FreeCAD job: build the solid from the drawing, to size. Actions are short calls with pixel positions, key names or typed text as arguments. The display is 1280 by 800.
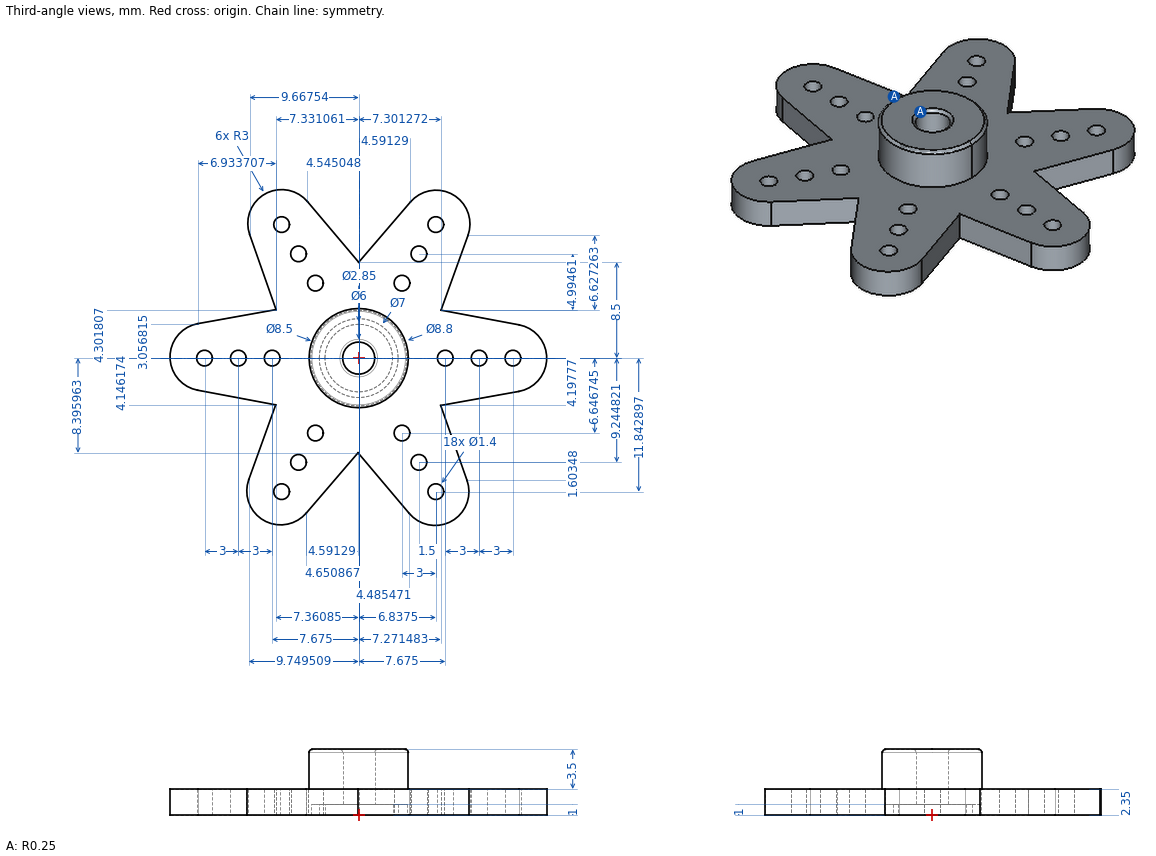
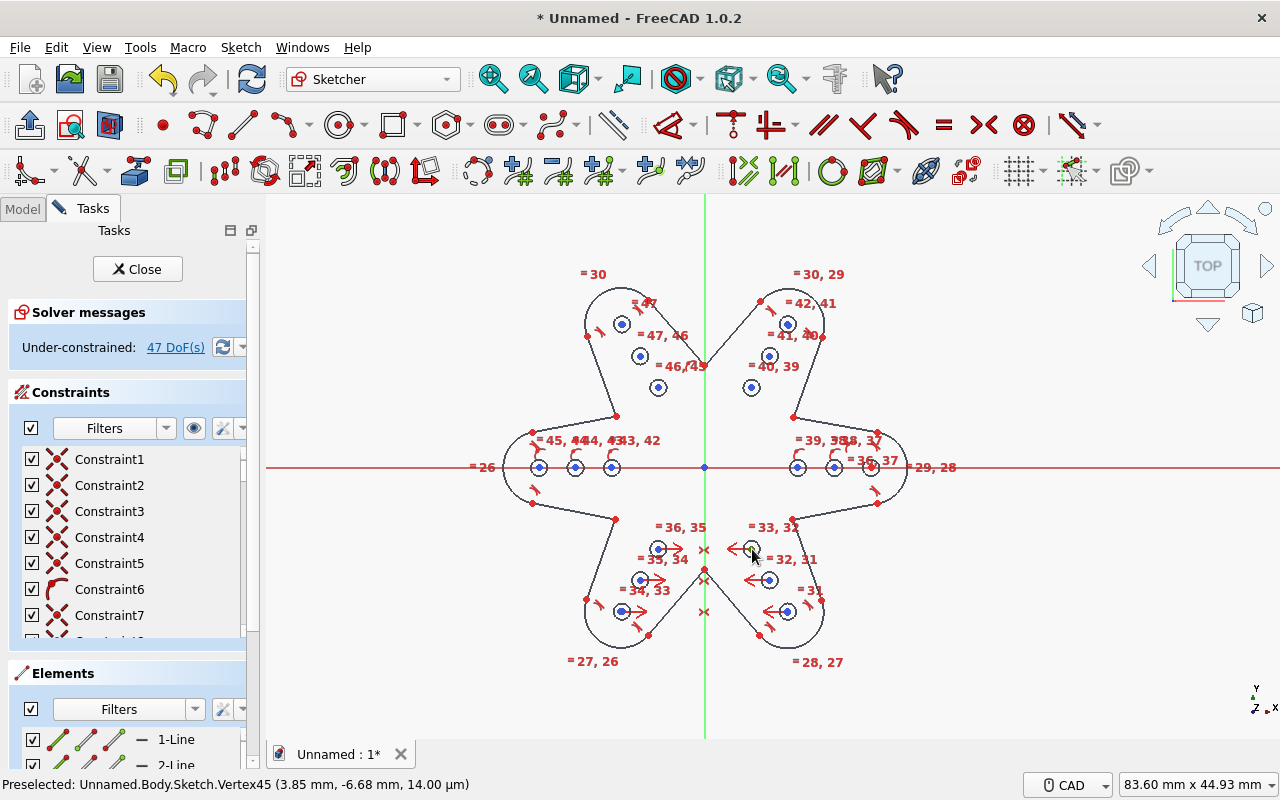
click(752, 388)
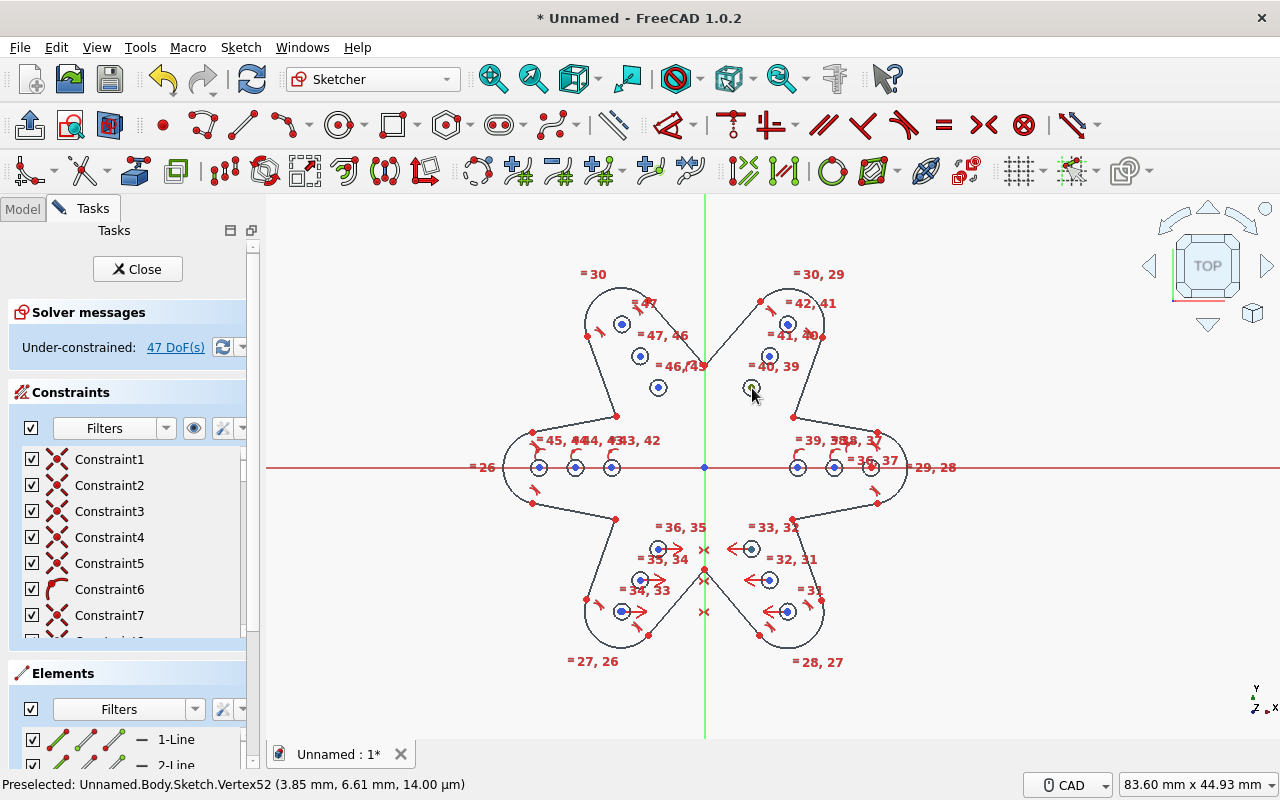
click(353, 468)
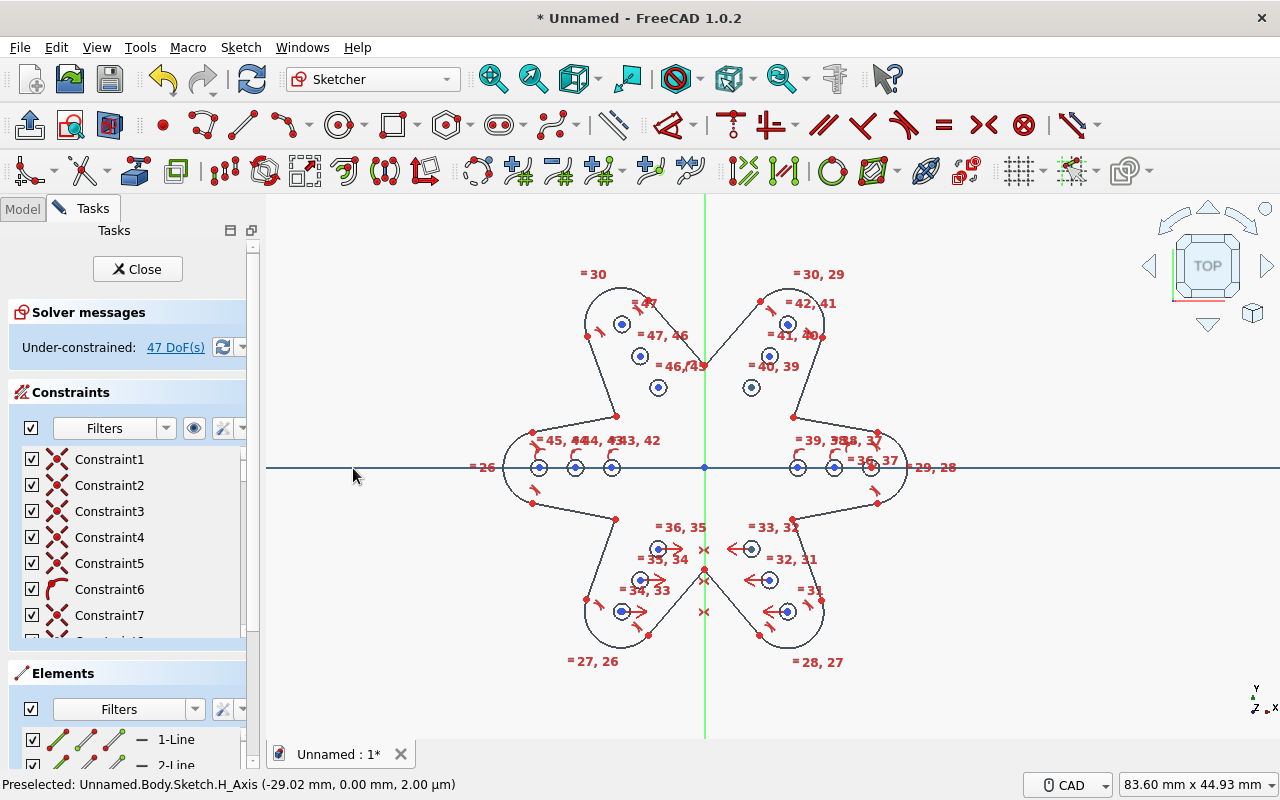
click(984, 126)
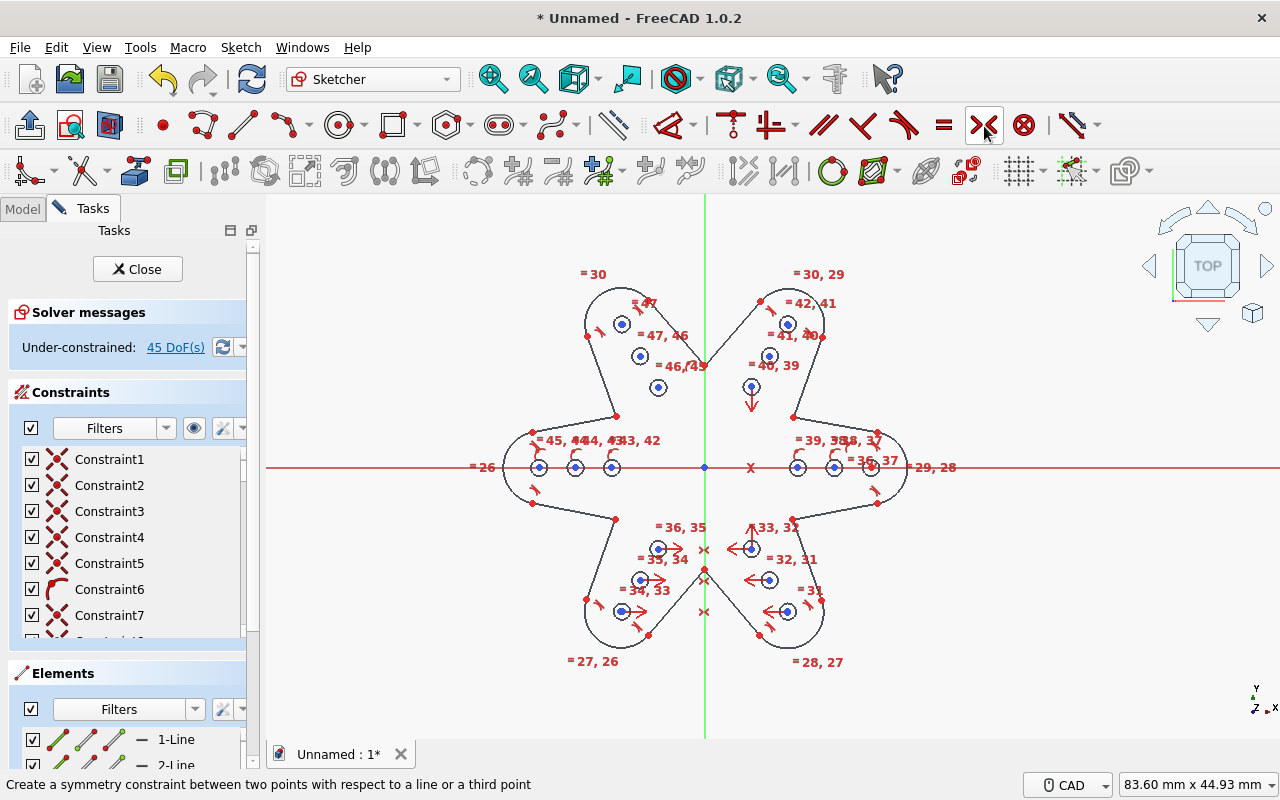
click(770, 580)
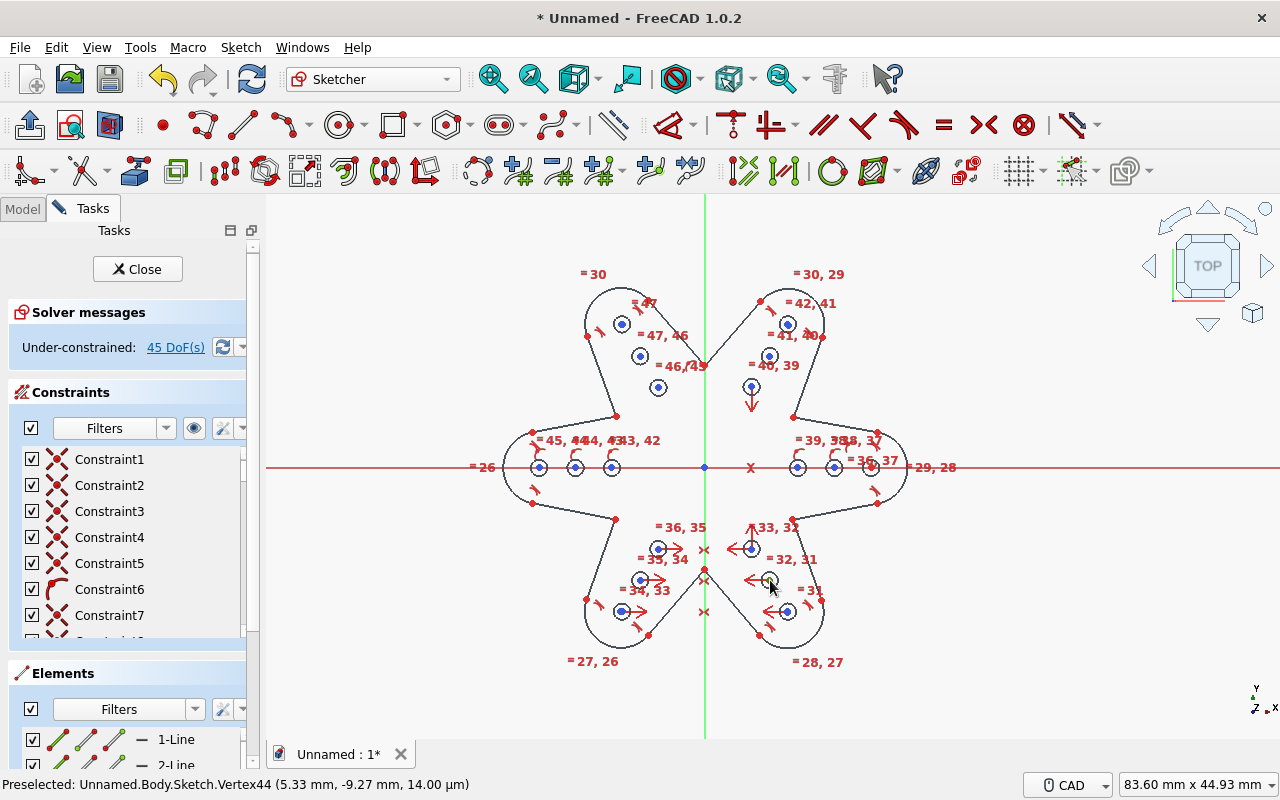
click(770, 356)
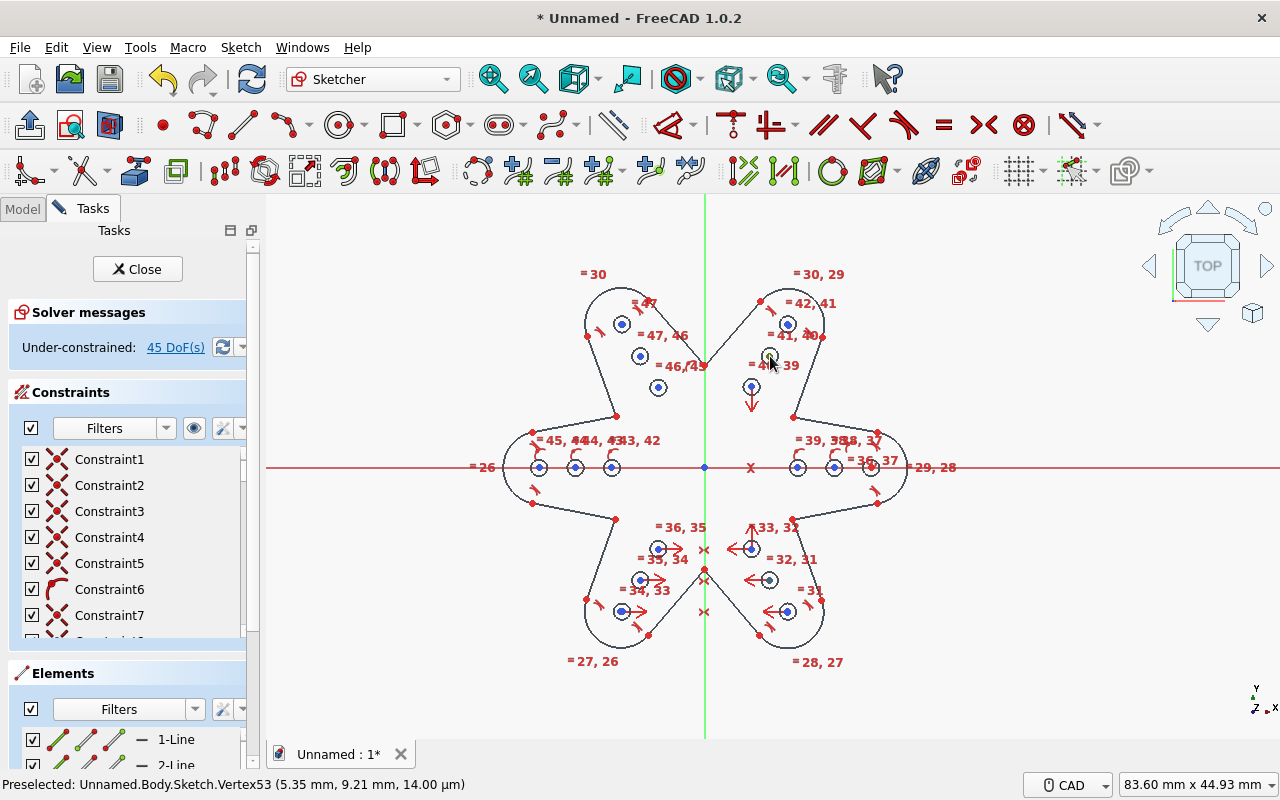
click(353, 468)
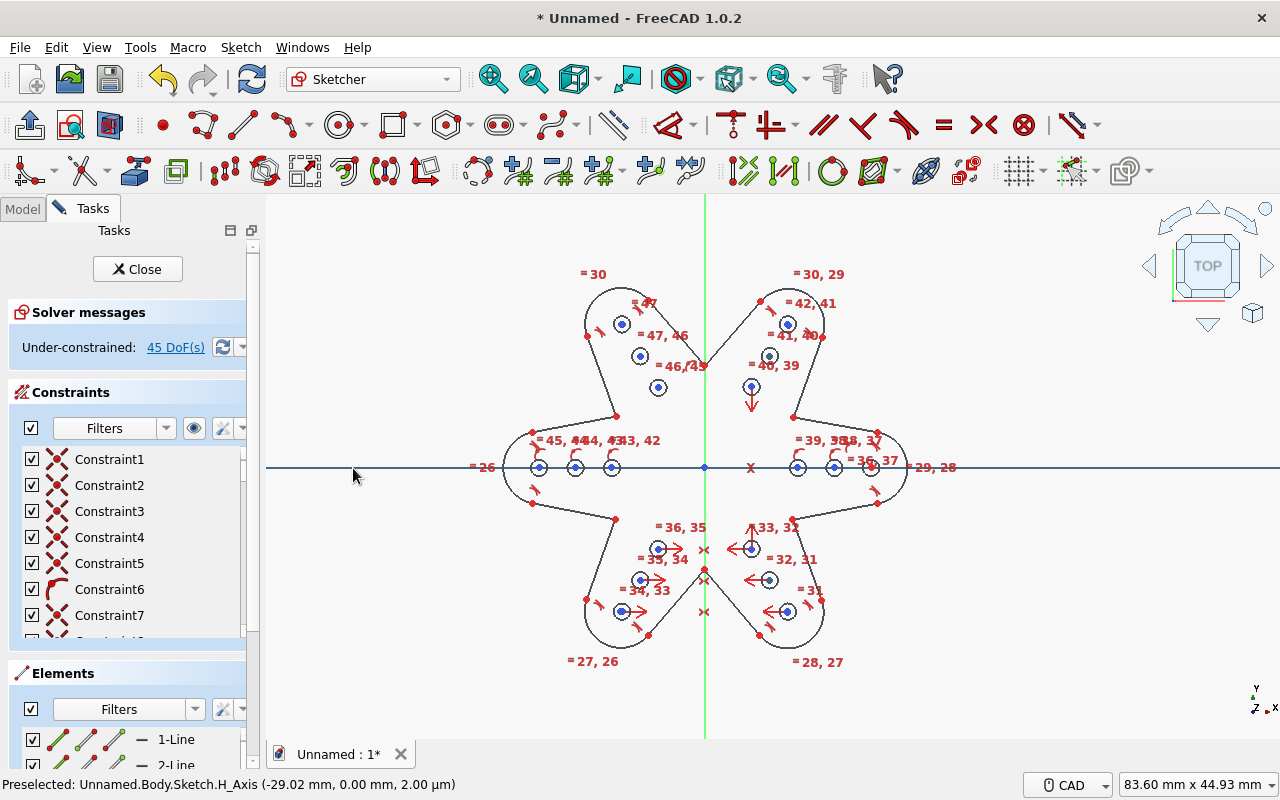
click(984, 126)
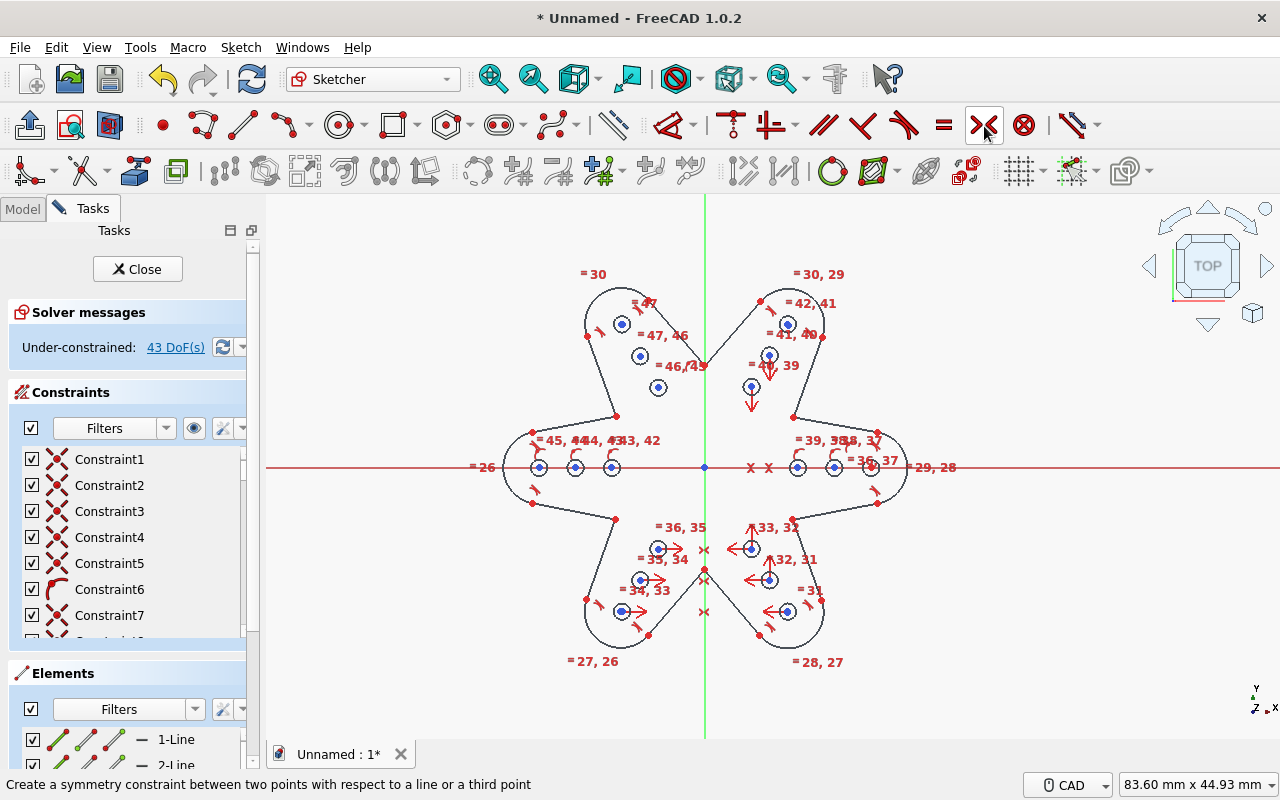
scroll(788, 612, up, 14)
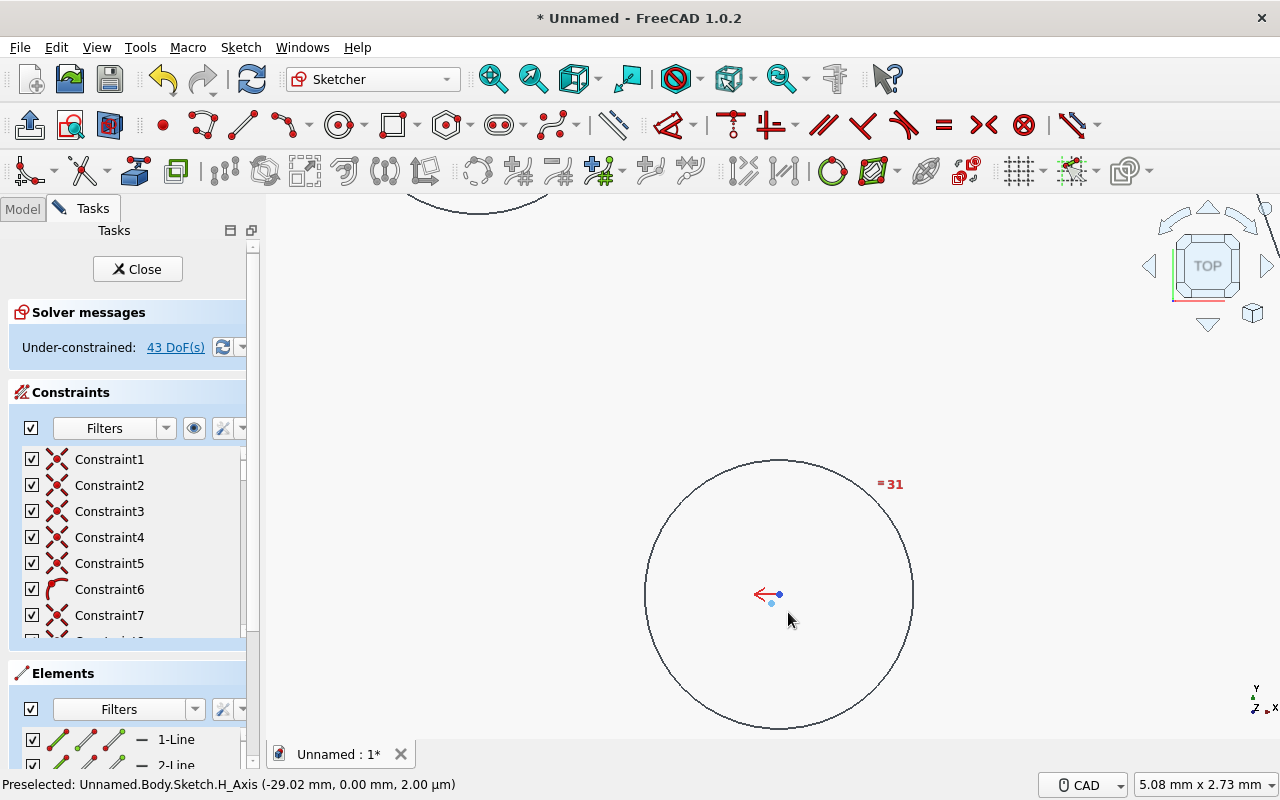
click(779, 594)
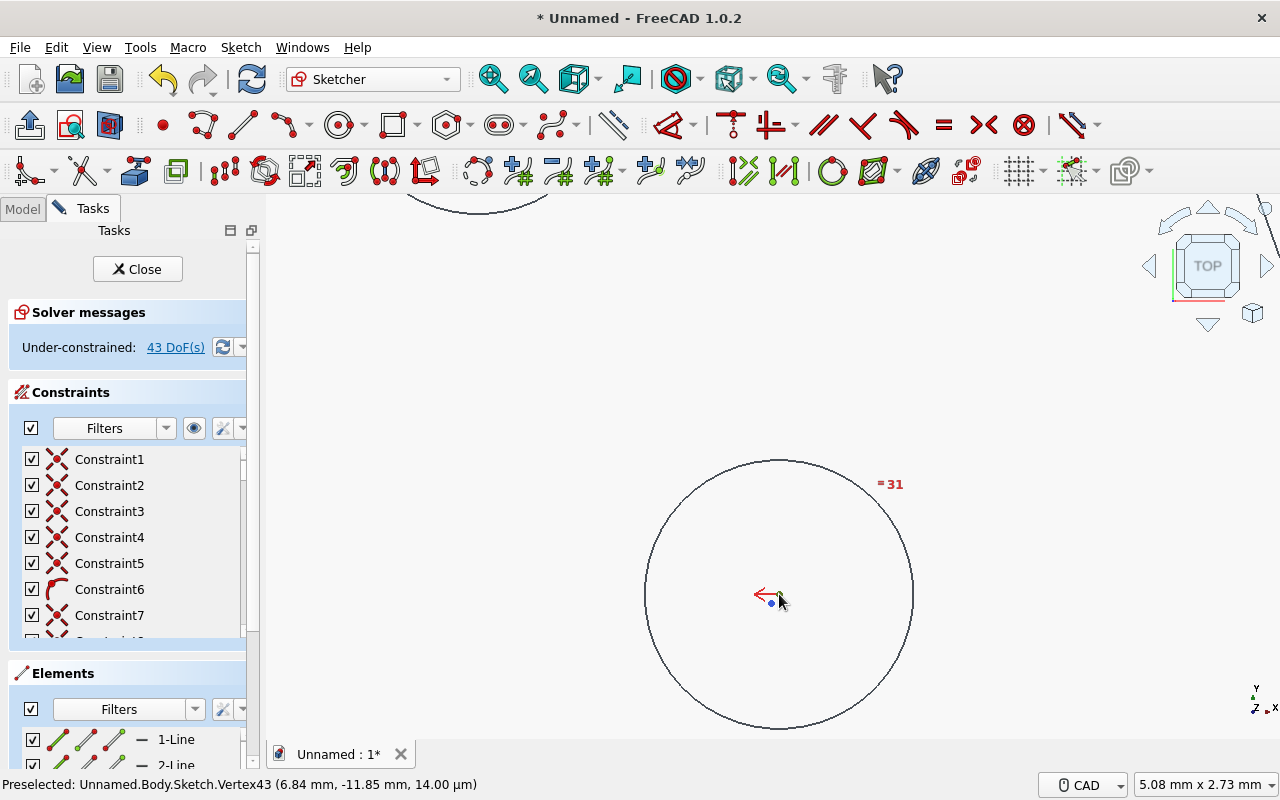
scroll(788, 612, down, 14)